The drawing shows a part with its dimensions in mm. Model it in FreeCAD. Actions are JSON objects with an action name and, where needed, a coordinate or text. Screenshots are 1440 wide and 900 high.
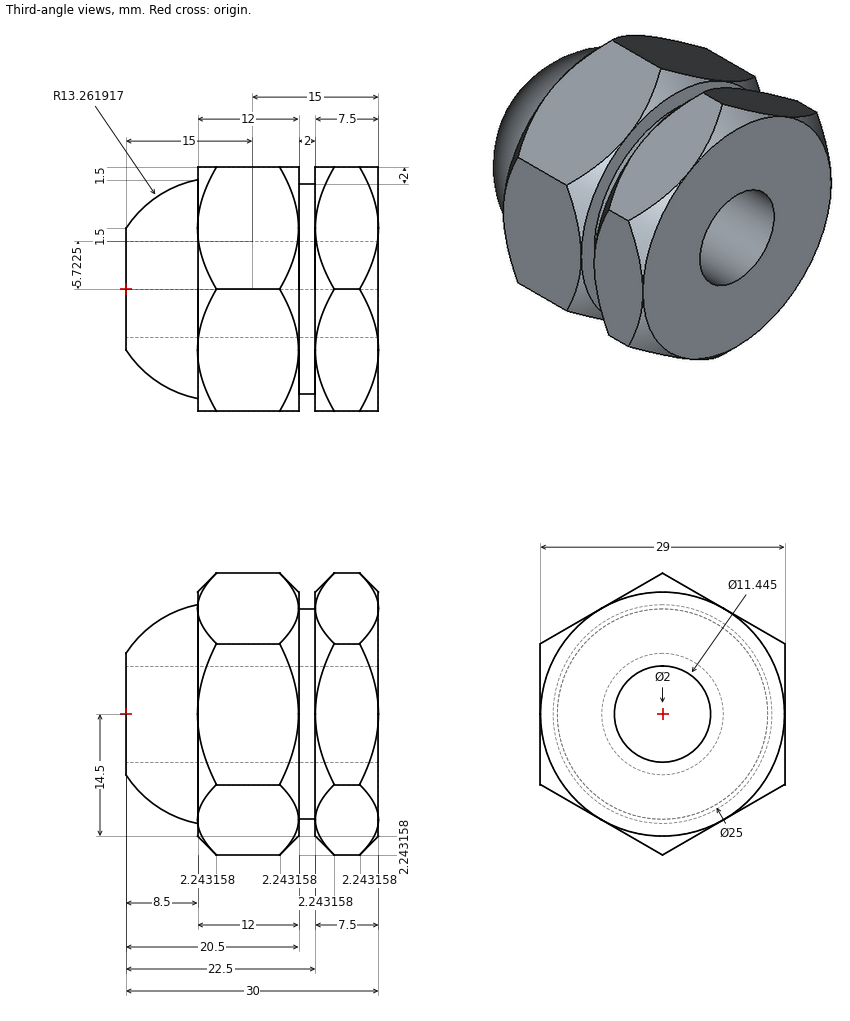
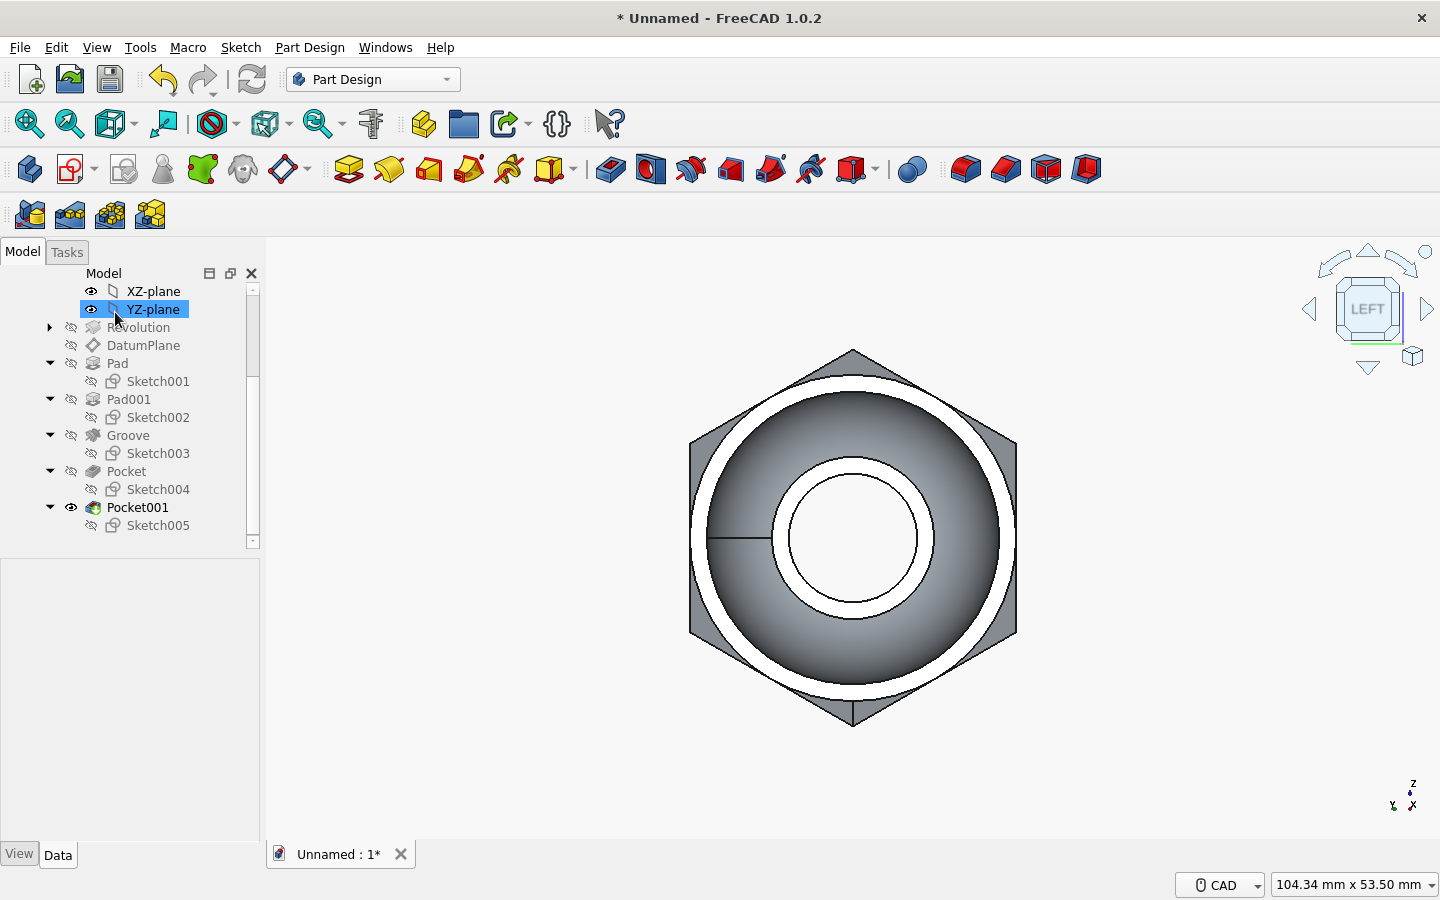
{"action": "key", "text": "0"}